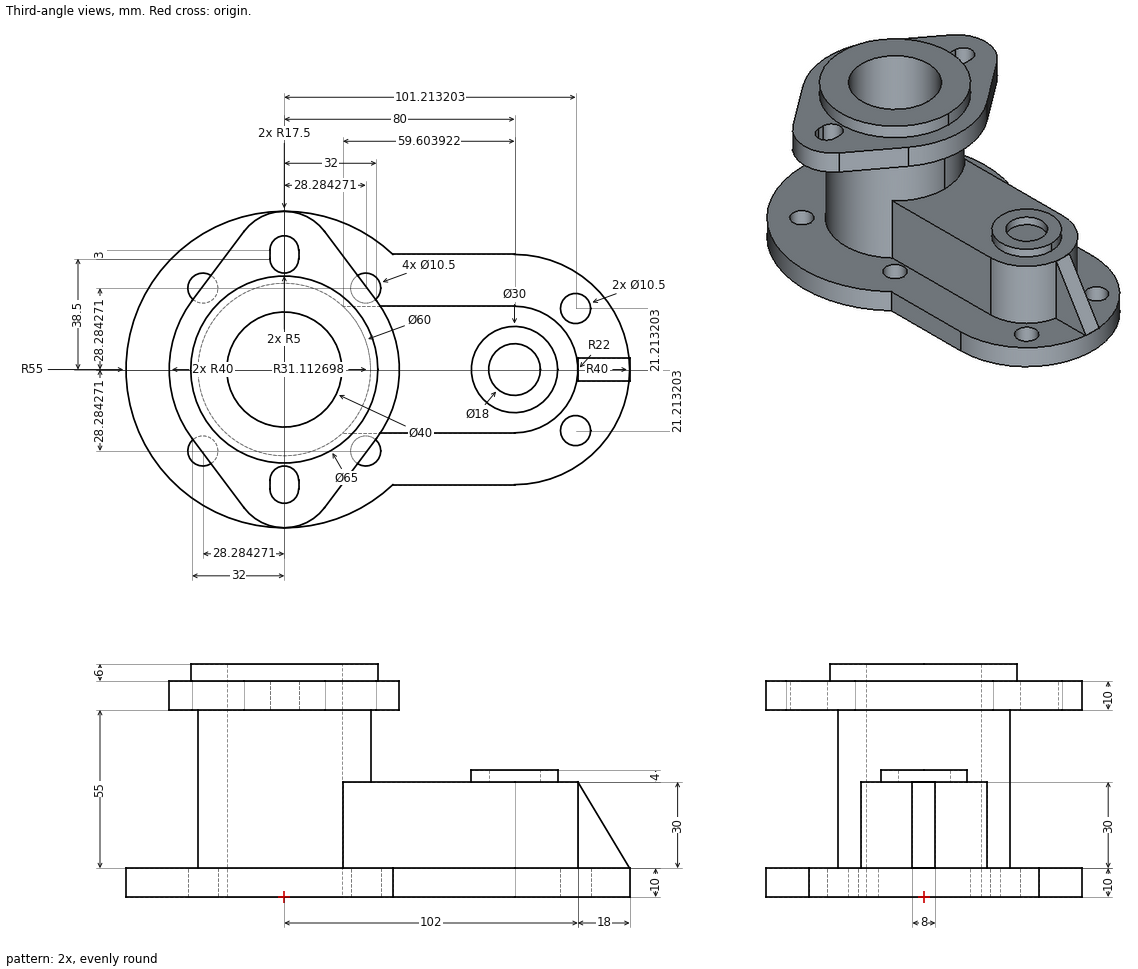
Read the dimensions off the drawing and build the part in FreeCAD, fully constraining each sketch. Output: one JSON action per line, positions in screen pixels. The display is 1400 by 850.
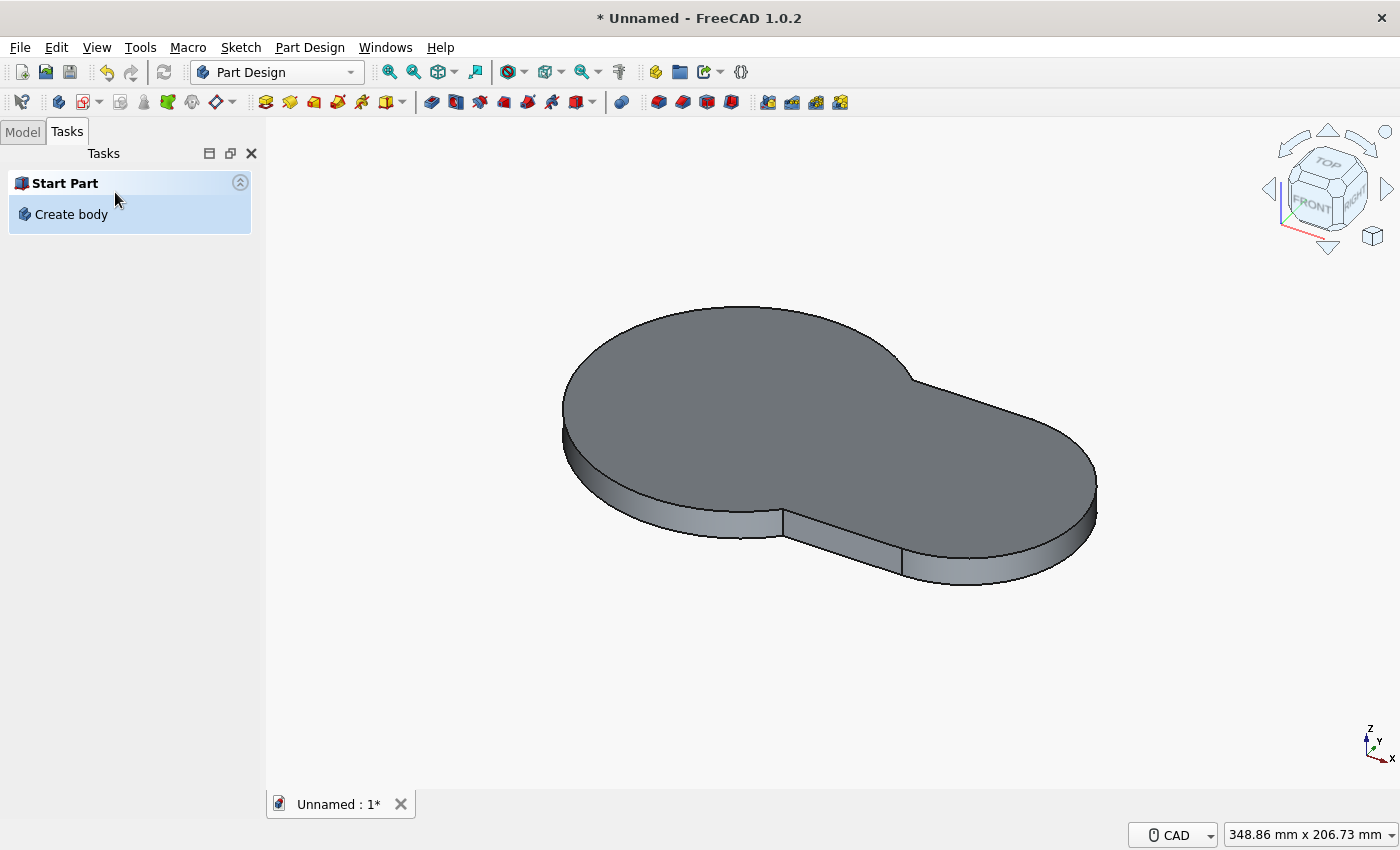
{"action": "left_click", "coordinate": [763, 415]}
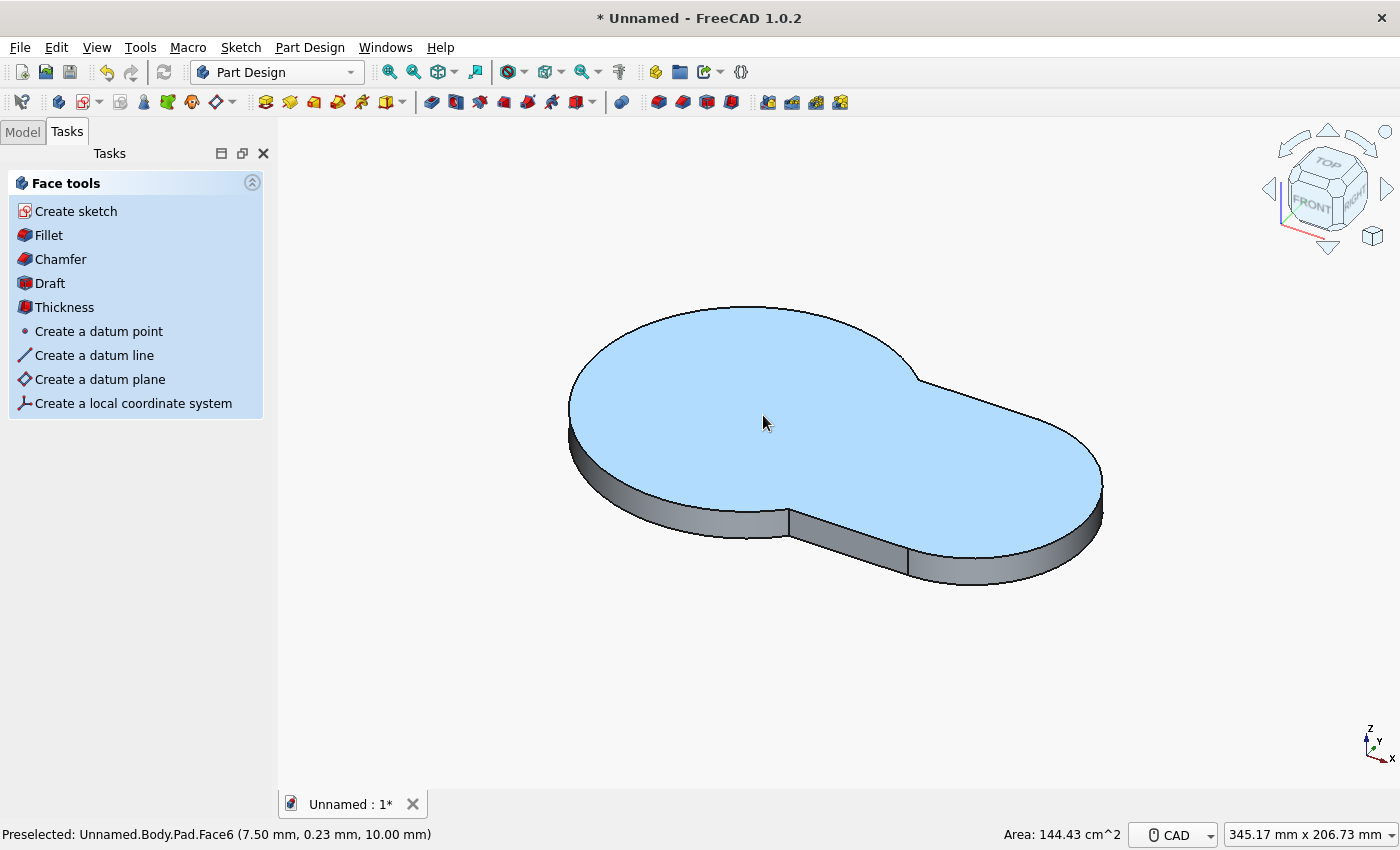
{"action": "left_click", "coordinate": [84, 102]}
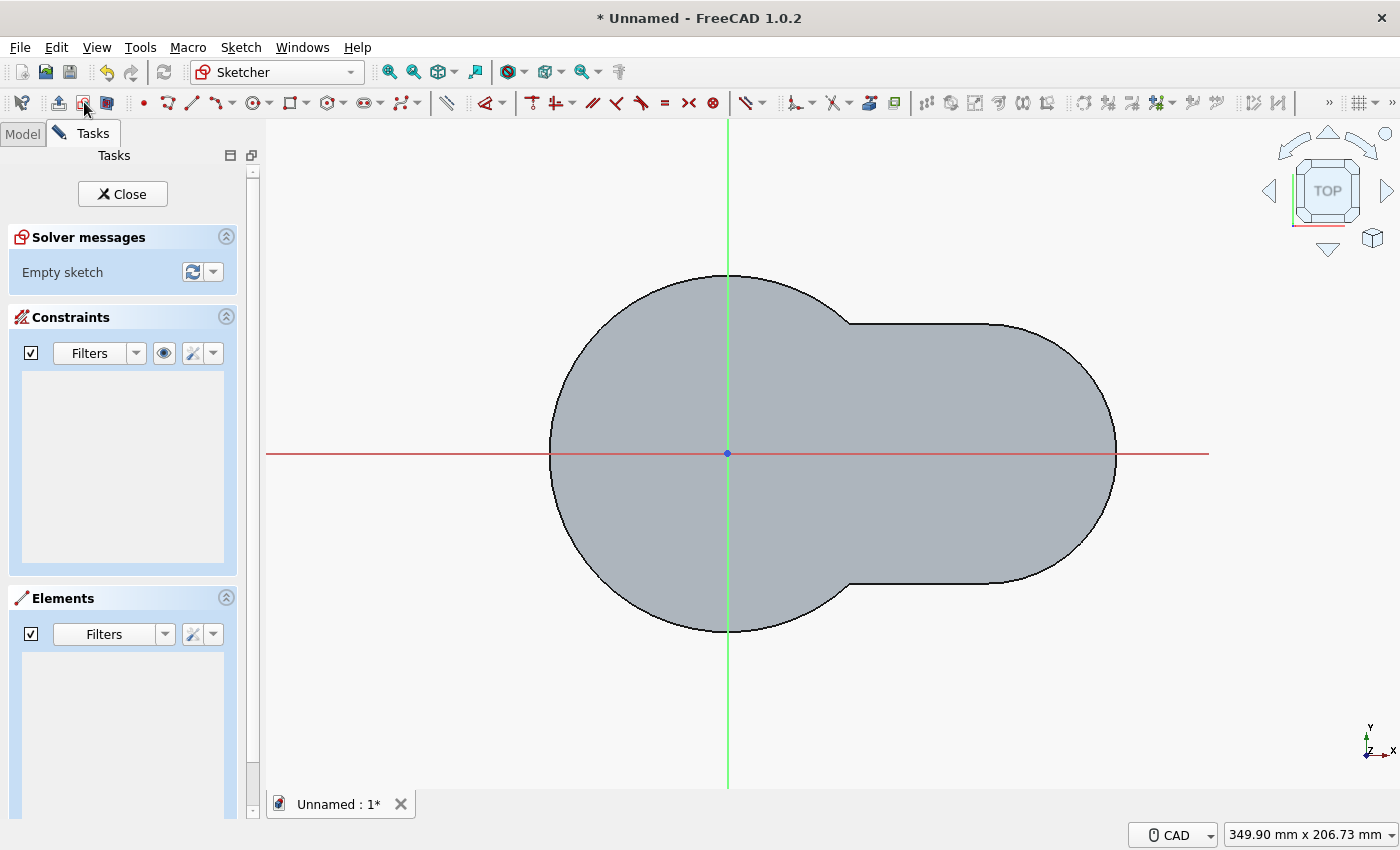
{"action": "scroll", "coordinate": [698, 454], "scroll_direction": "up", "scroll_amount": 4}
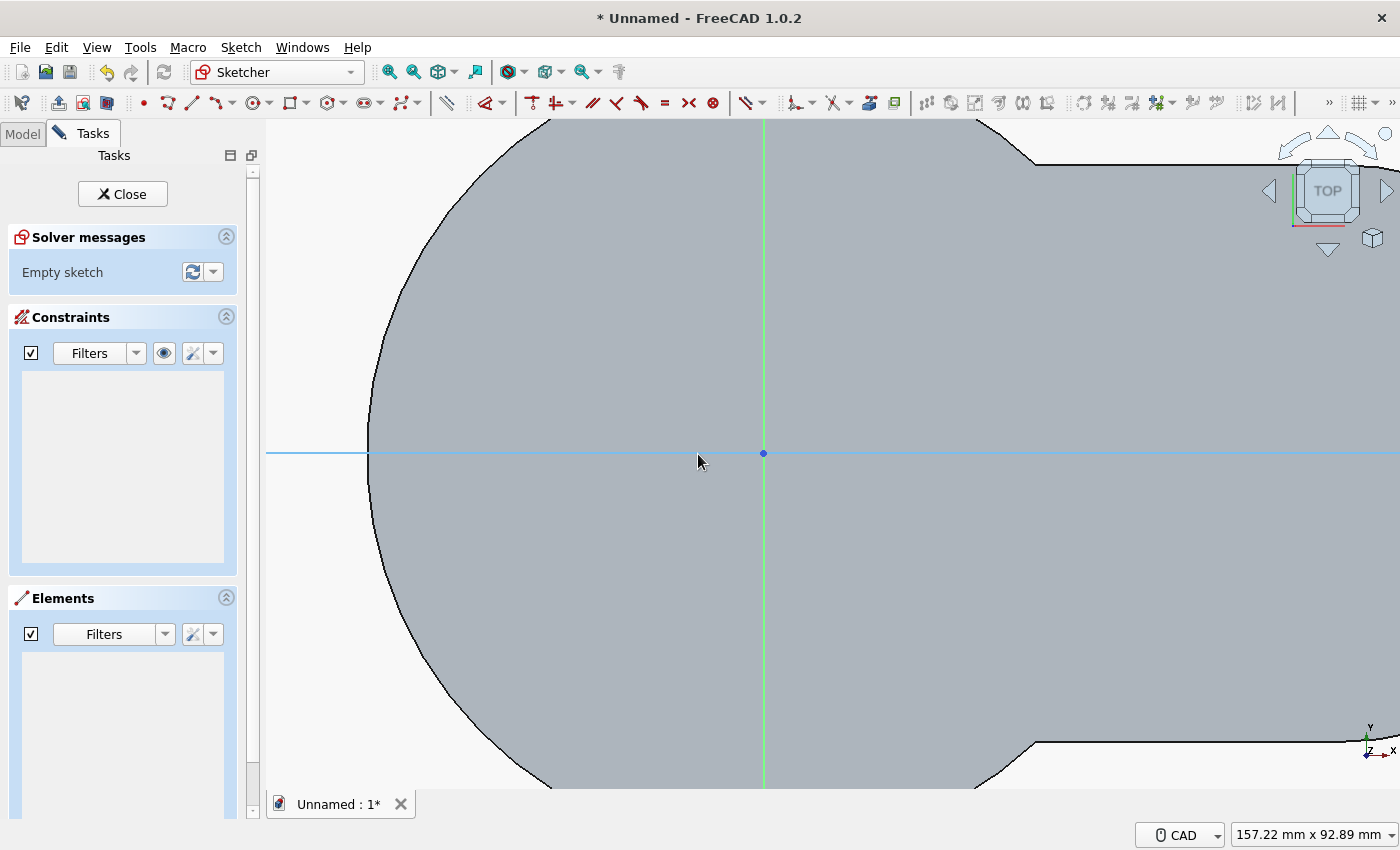
{"action": "left_click", "coordinate": [254, 104]}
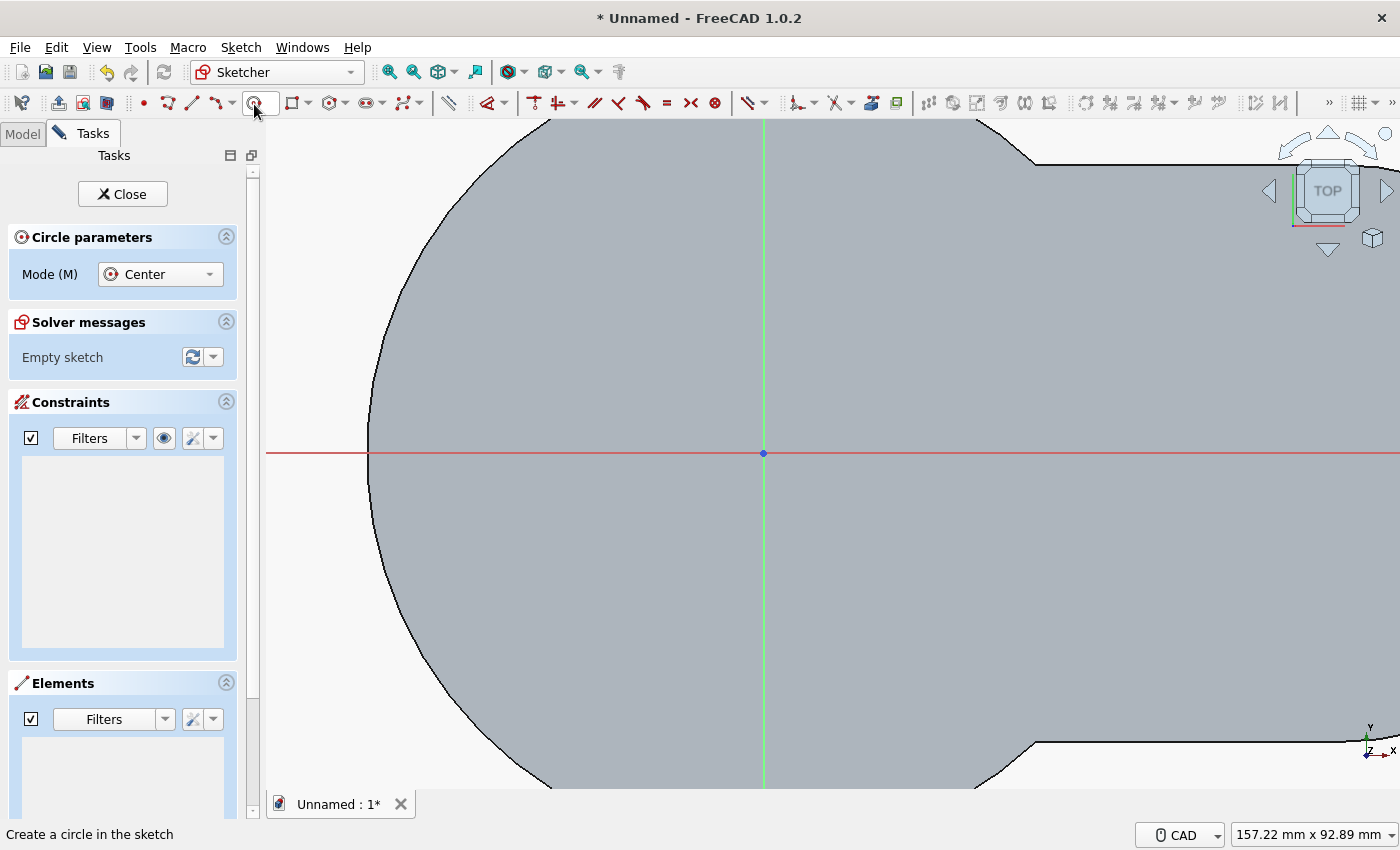
{"action": "left_click", "coordinate": [764, 453]}
{"action": "mouse_move", "coordinate": [917, 300]}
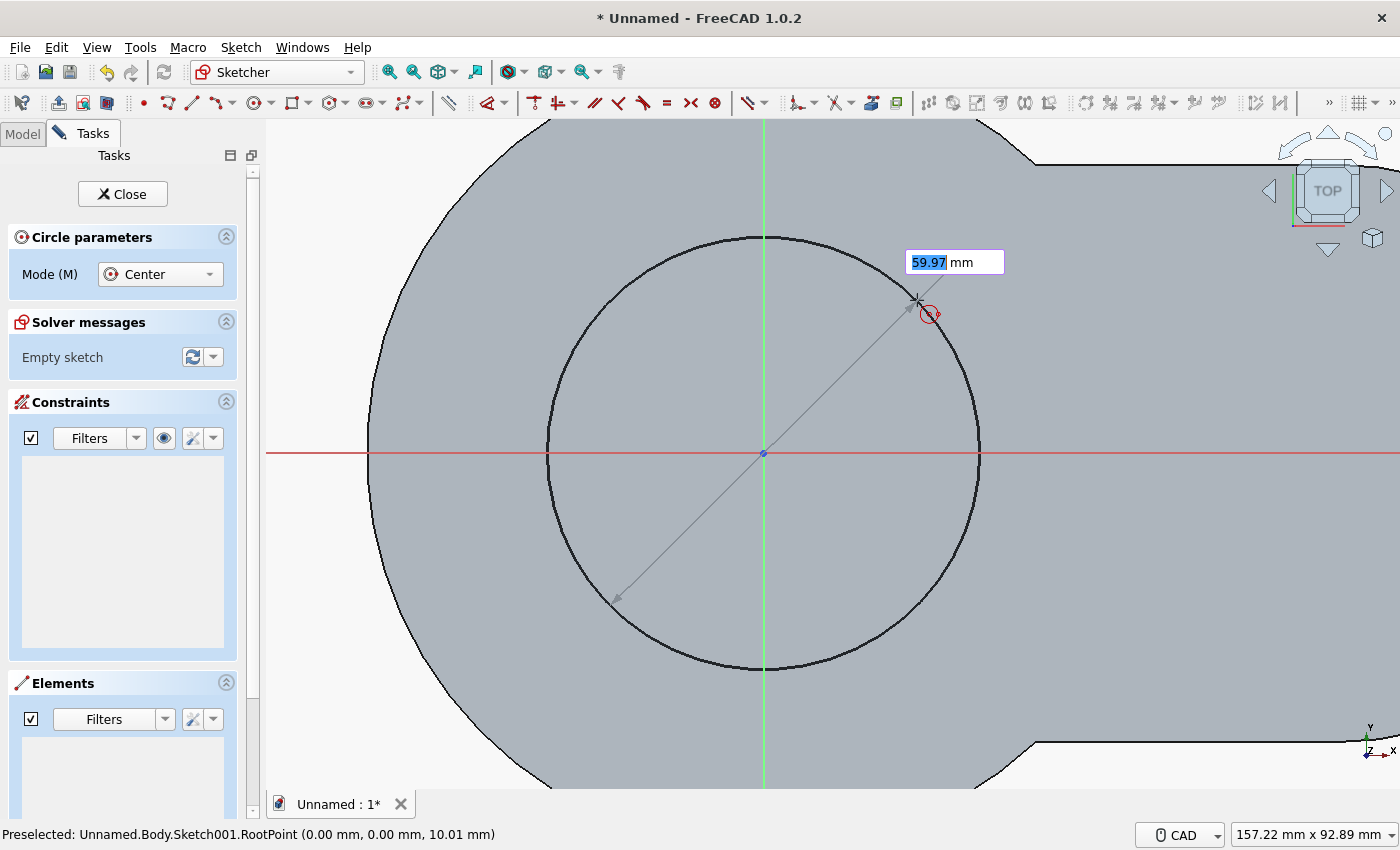
{"action": "type", "text": "60"}
{"action": "key", "text": "Return"}
{"action": "key", "text": "Escape"}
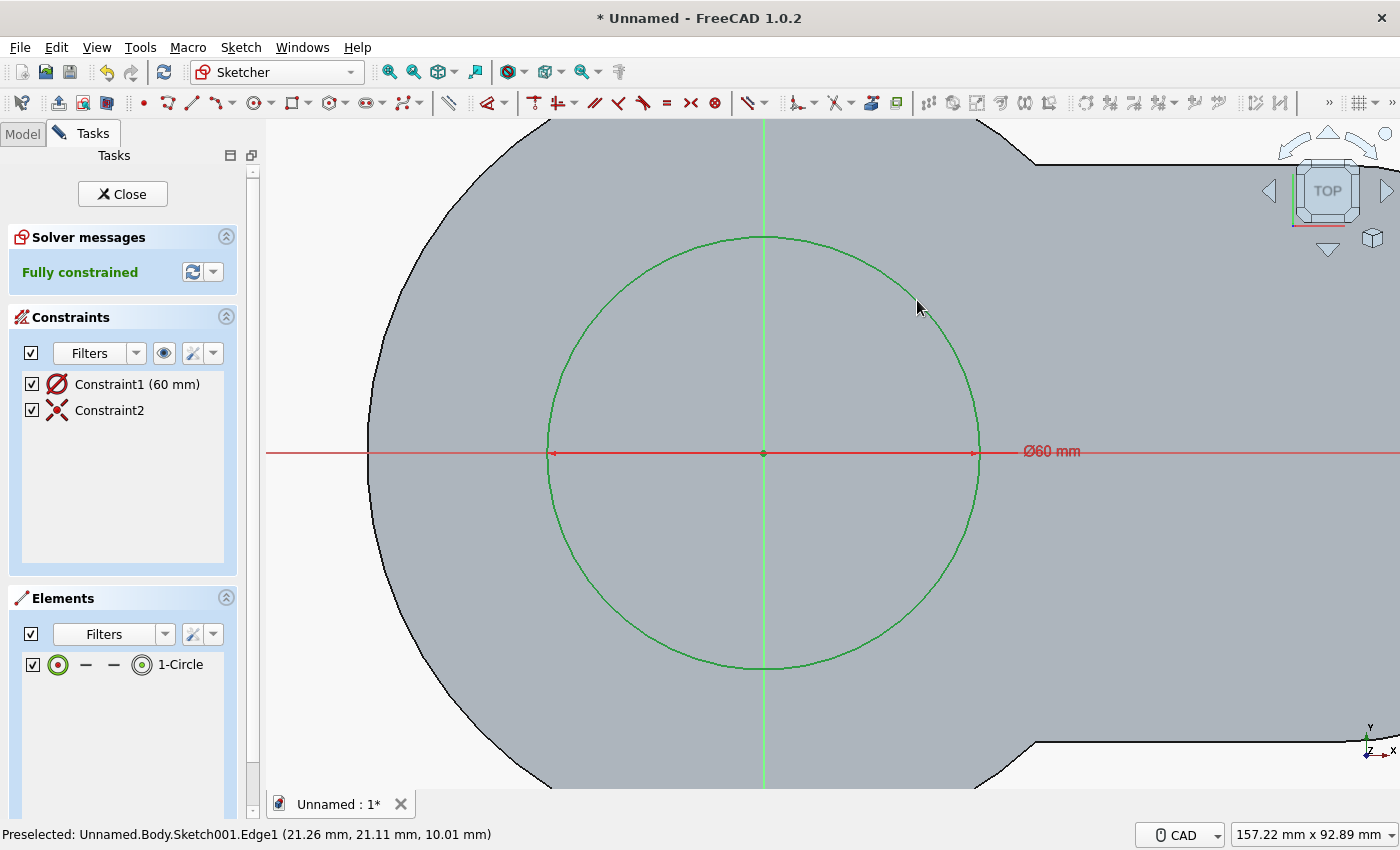
{"action": "left_click", "coordinate": [123, 194]}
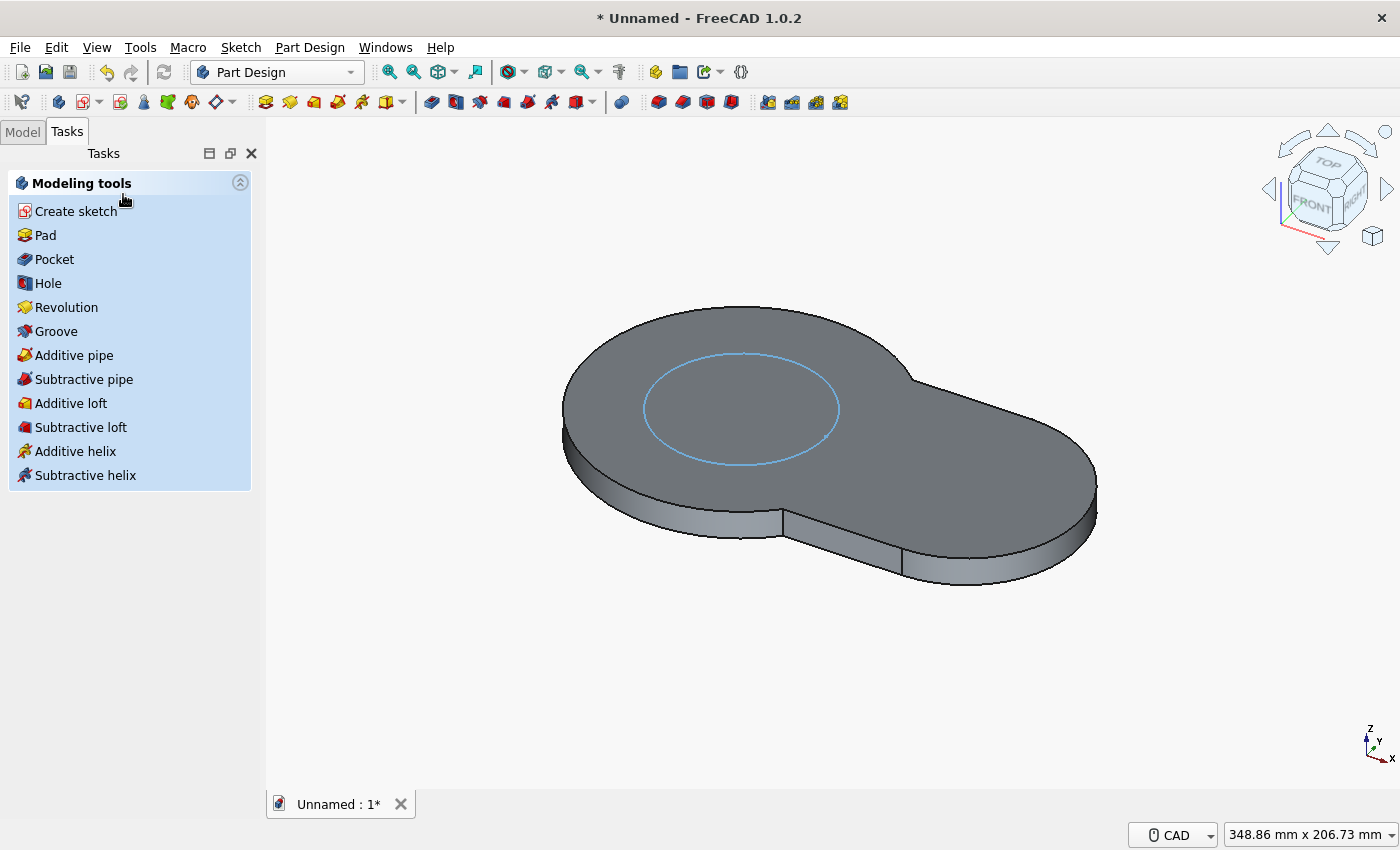
{"action": "left_click", "coordinate": [266, 102]}